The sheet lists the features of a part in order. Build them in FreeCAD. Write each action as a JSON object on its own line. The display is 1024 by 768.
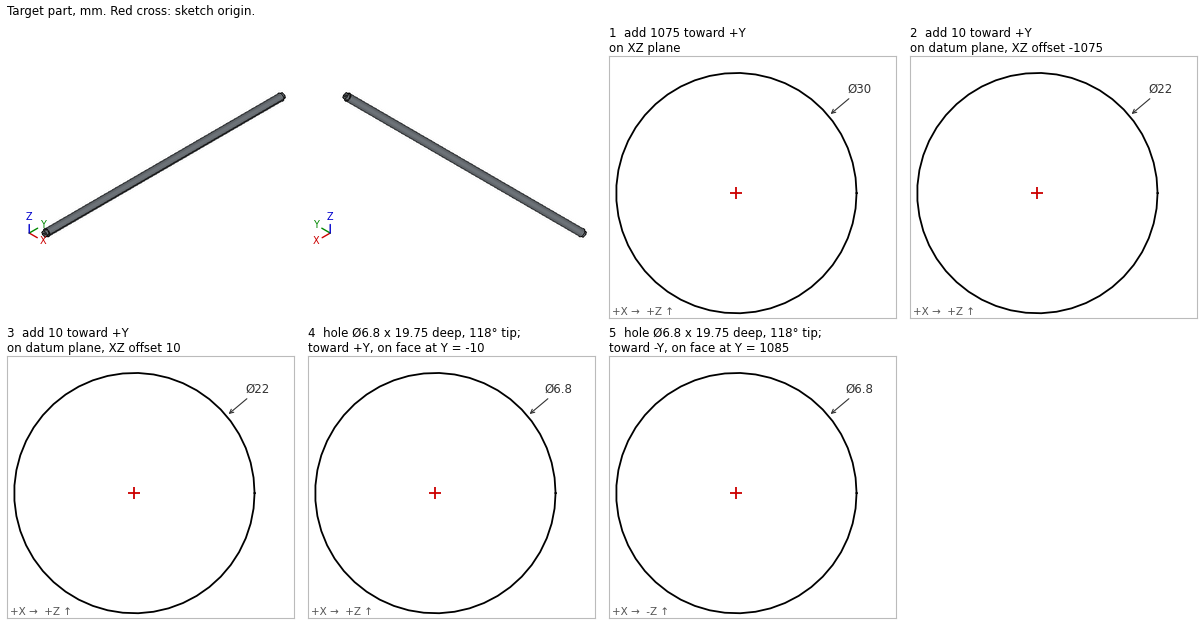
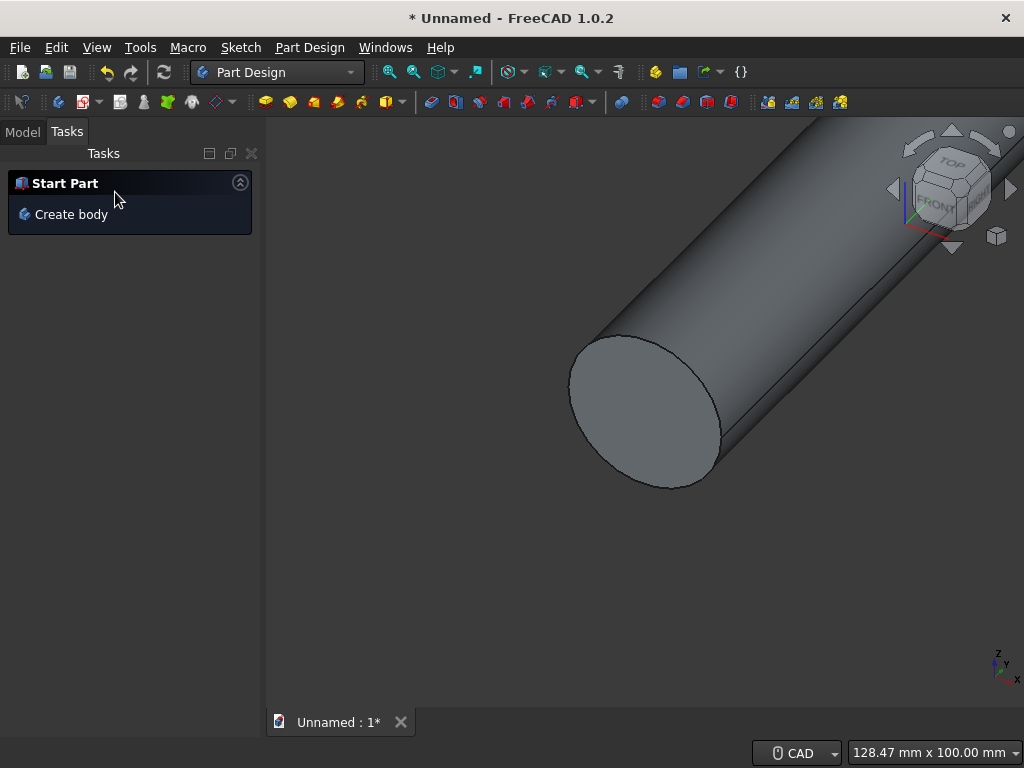
{"action": "left_click", "coordinate": [390, 72]}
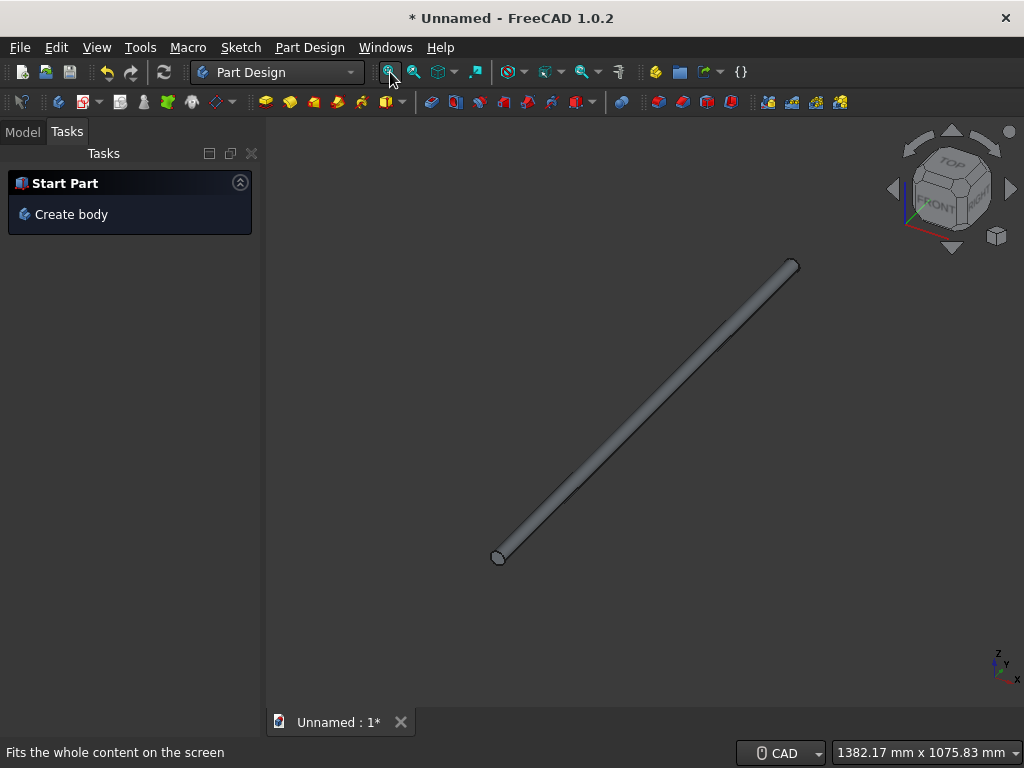
{"action": "key", "text": "4"}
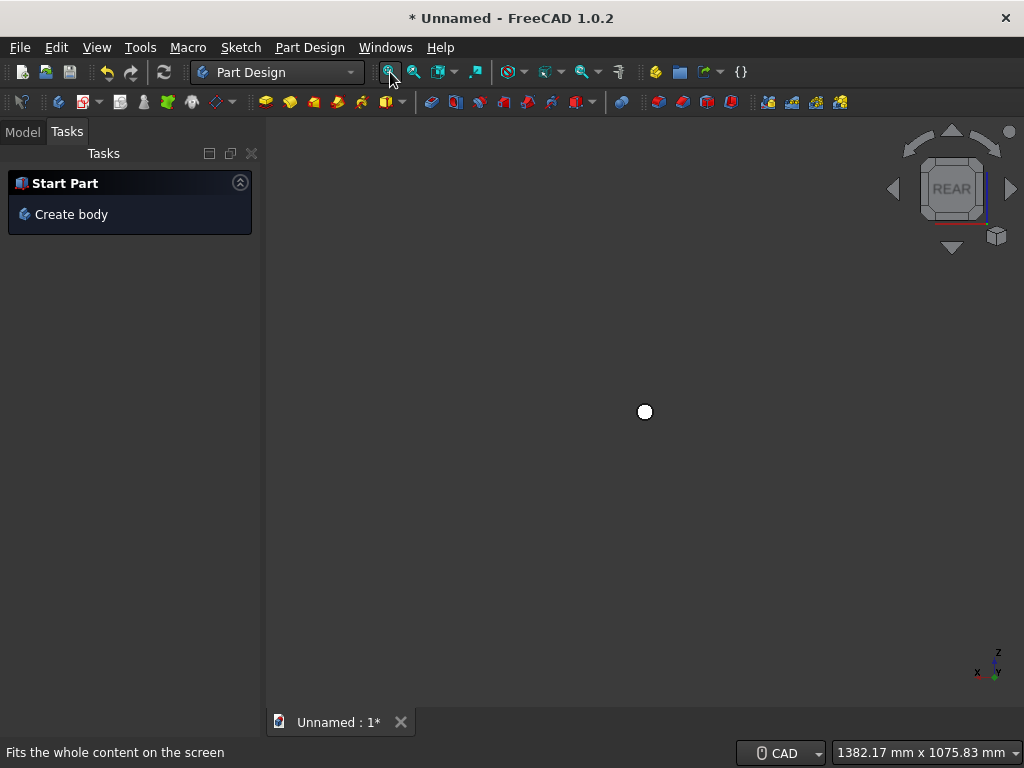
{"action": "left_click", "coordinate": [390, 72]}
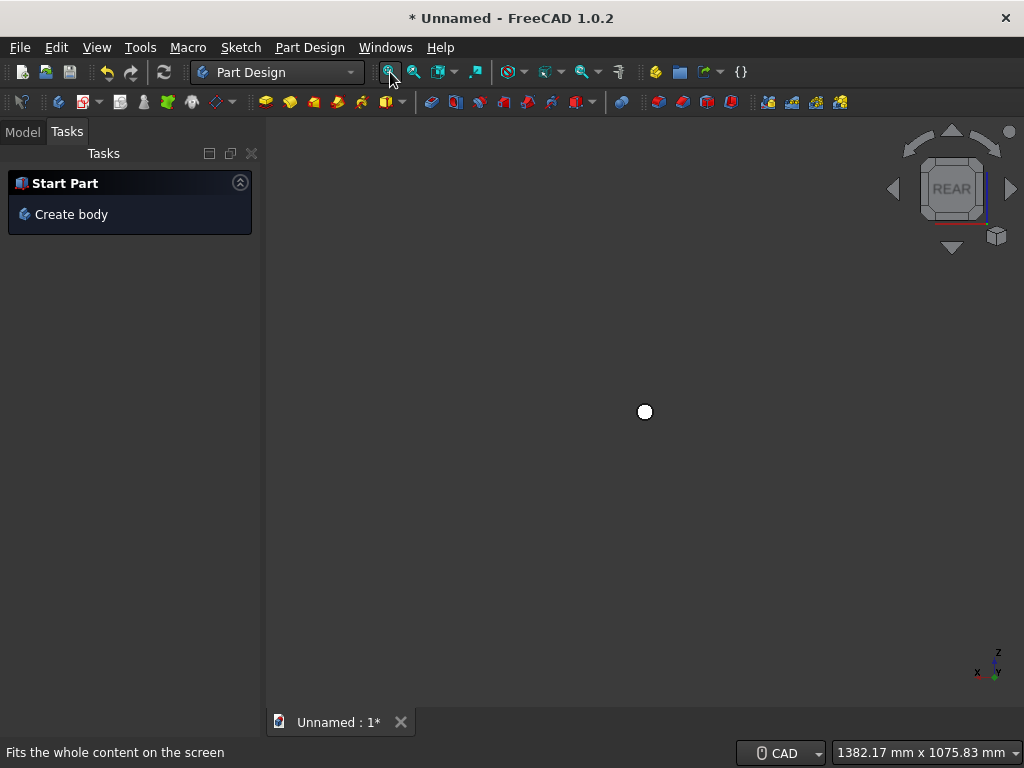
{"action": "key", "text": "5"}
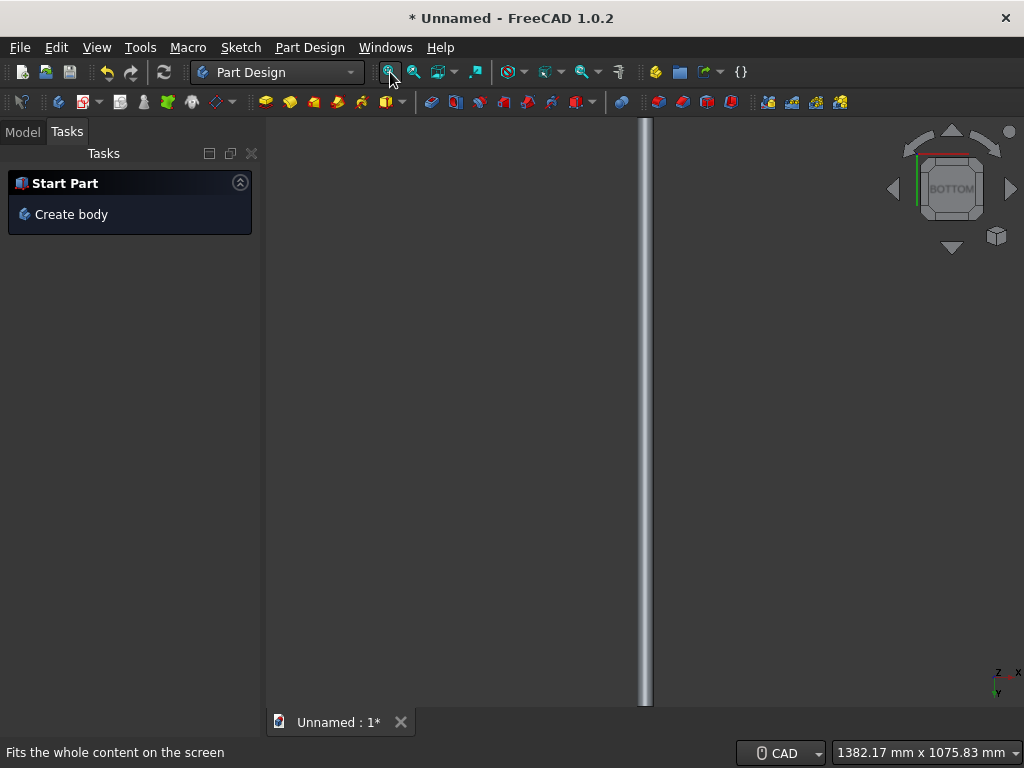
{"action": "left_click", "coordinate": [390, 72]}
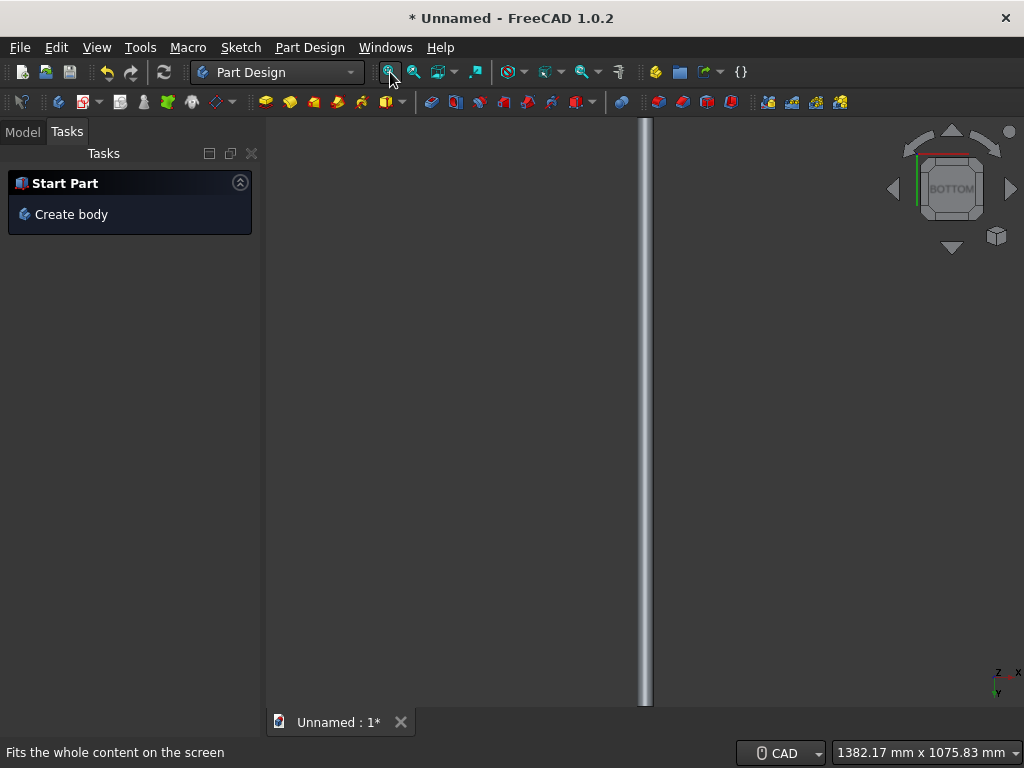
{"action": "key", "text": "3"}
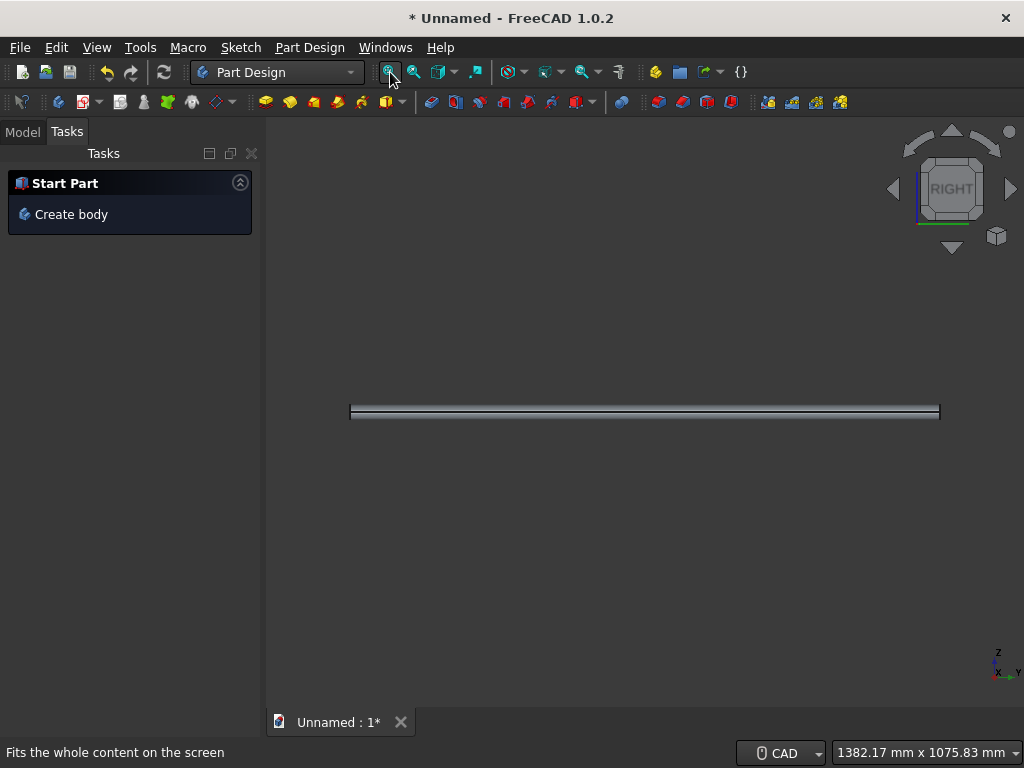
{"action": "left_click", "coordinate": [23, 131]}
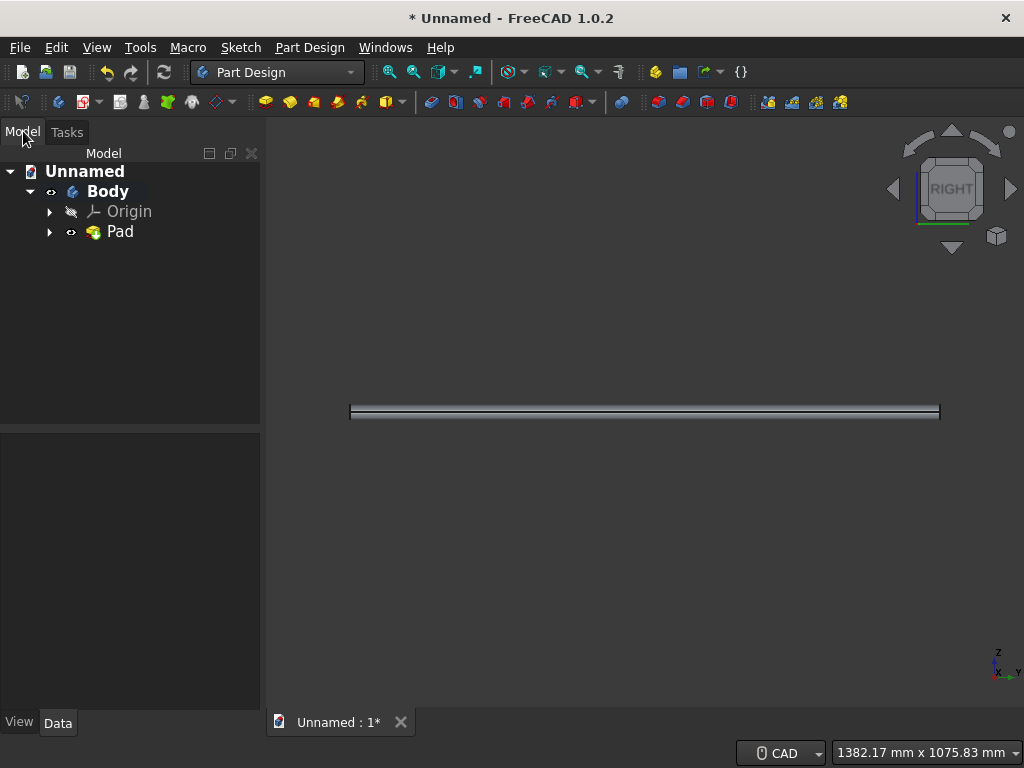
{"action": "left_click", "coordinate": [50, 212]}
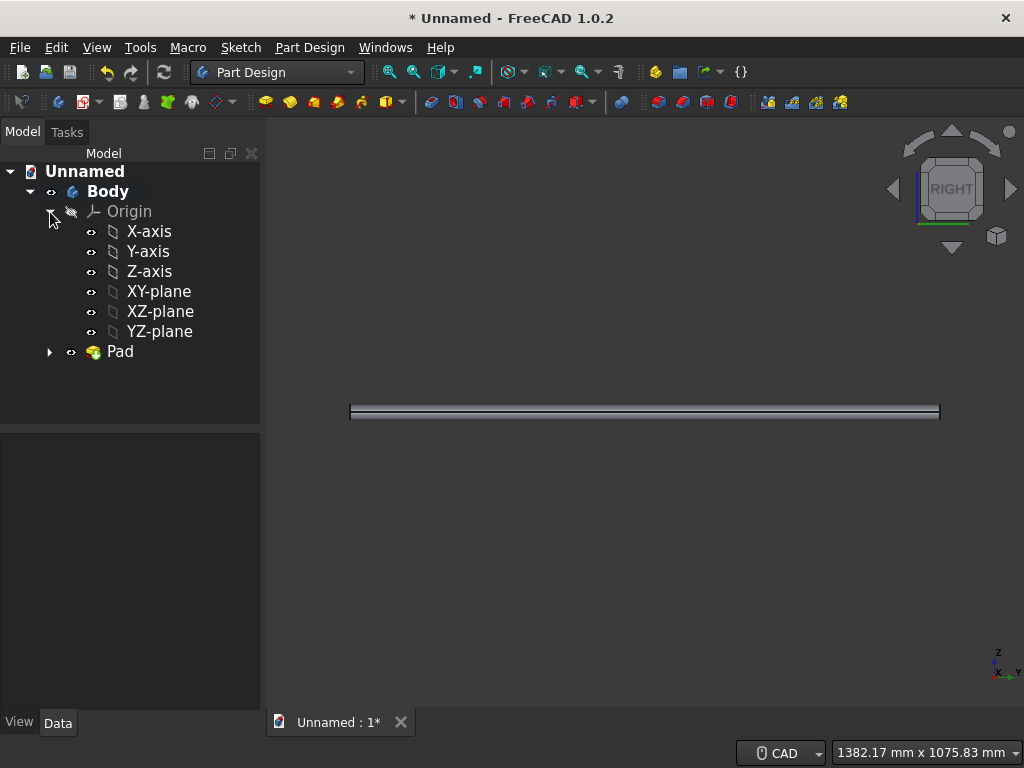
{"action": "left_click", "coordinate": [136, 312]}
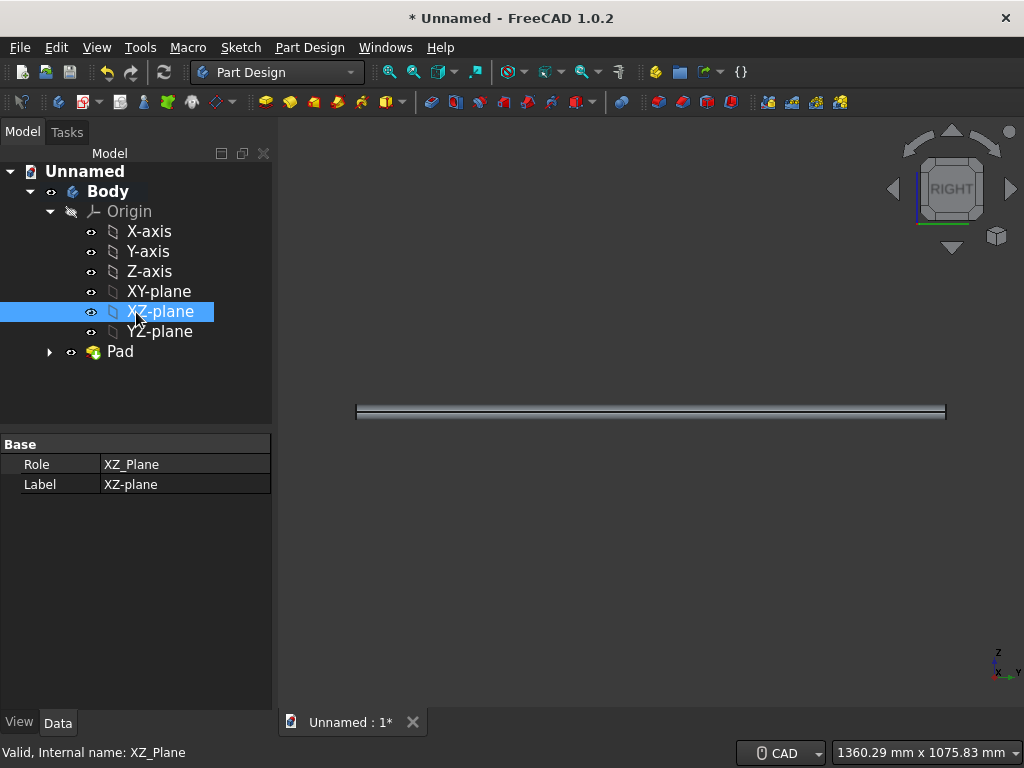
{"action": "left_click", "coordinate": [216, 102]}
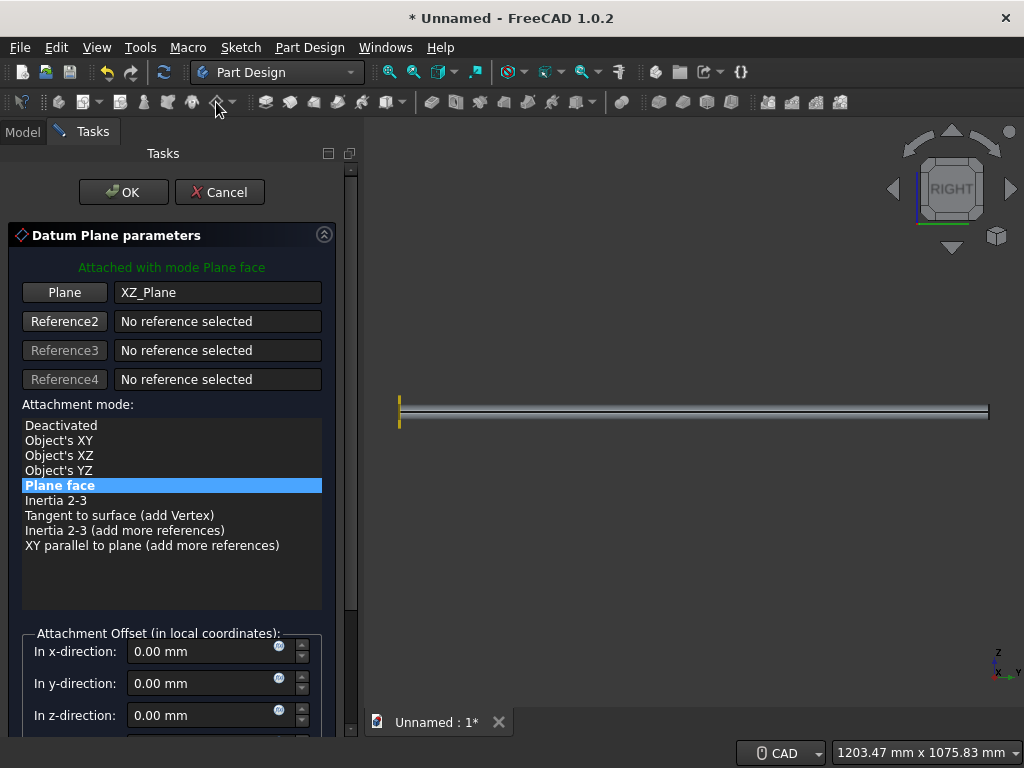
{"action": "triple_click", "coordinate": [210, 715]}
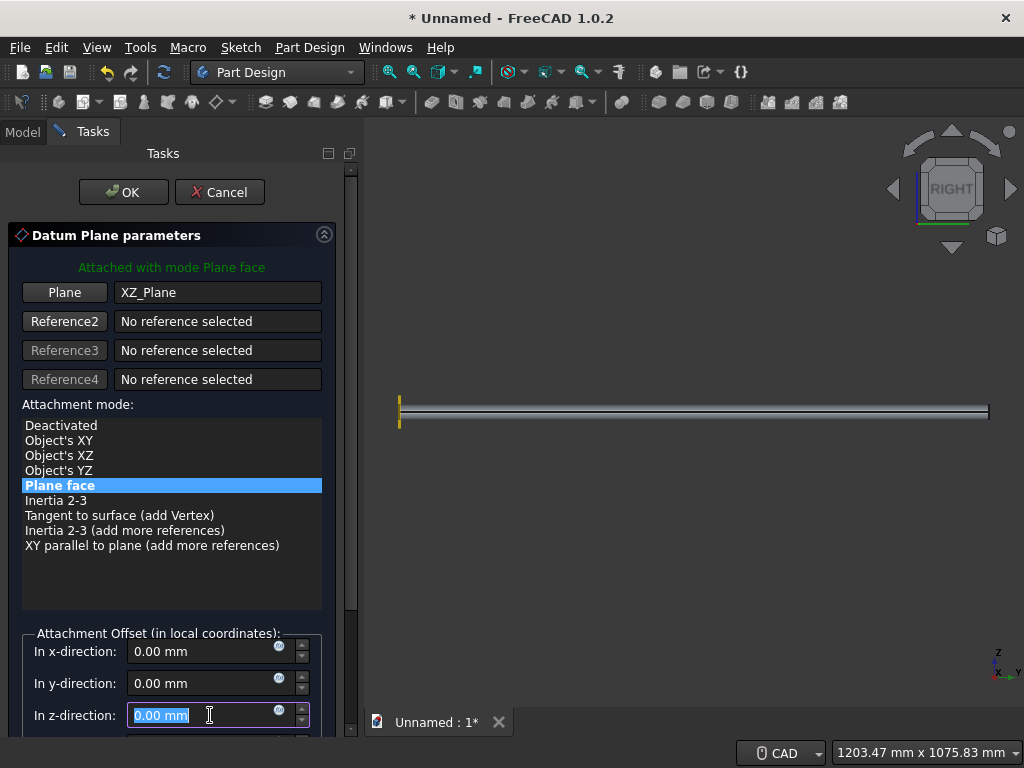
{"action": "type", "text": "-1075"}
{"action": "key", "text": "Tab"}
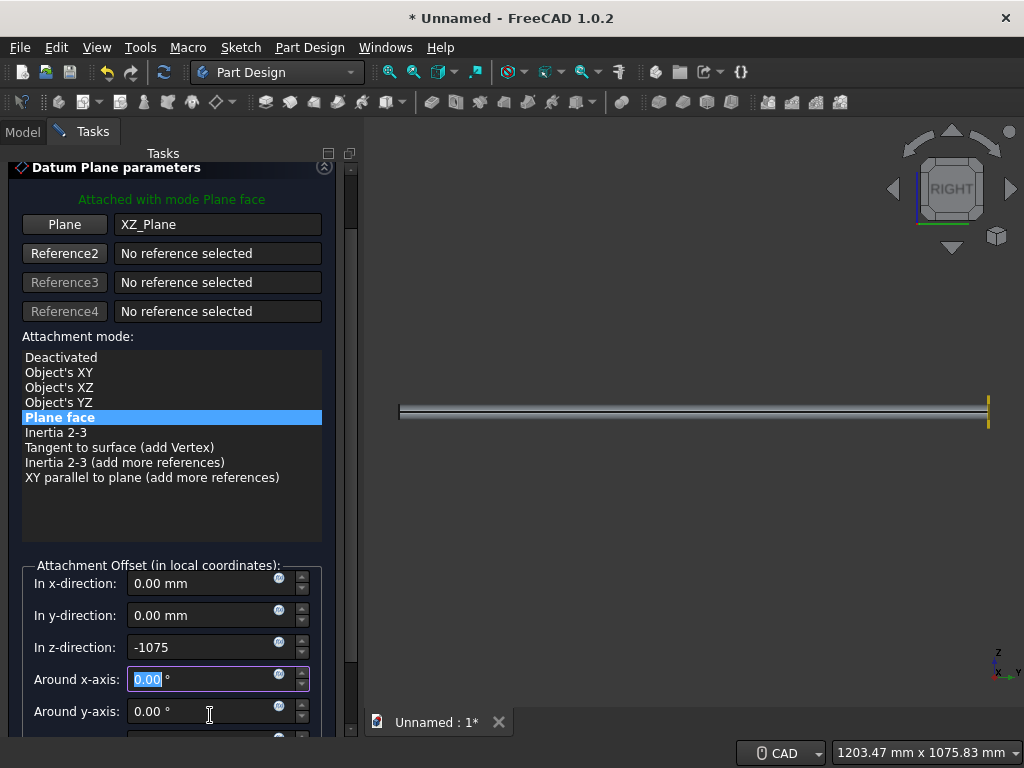
{"action": "scroll", "coordinate": [351, 450], "scroll_direction": "up", "scroll_amount": 2}